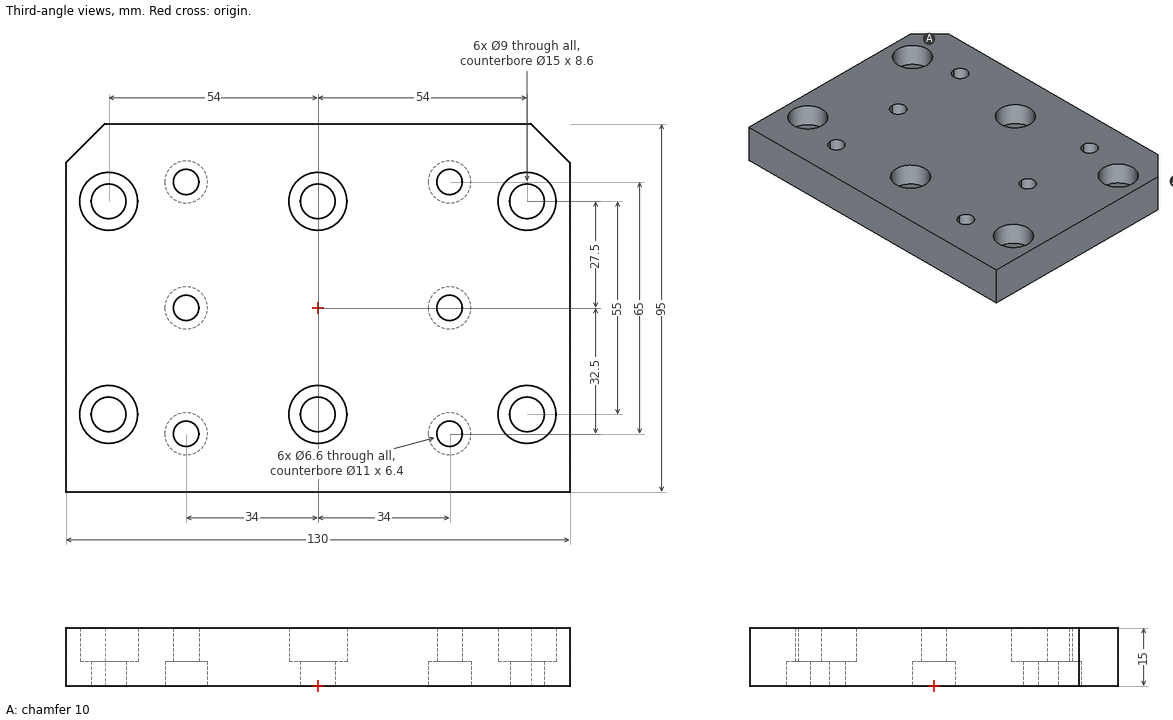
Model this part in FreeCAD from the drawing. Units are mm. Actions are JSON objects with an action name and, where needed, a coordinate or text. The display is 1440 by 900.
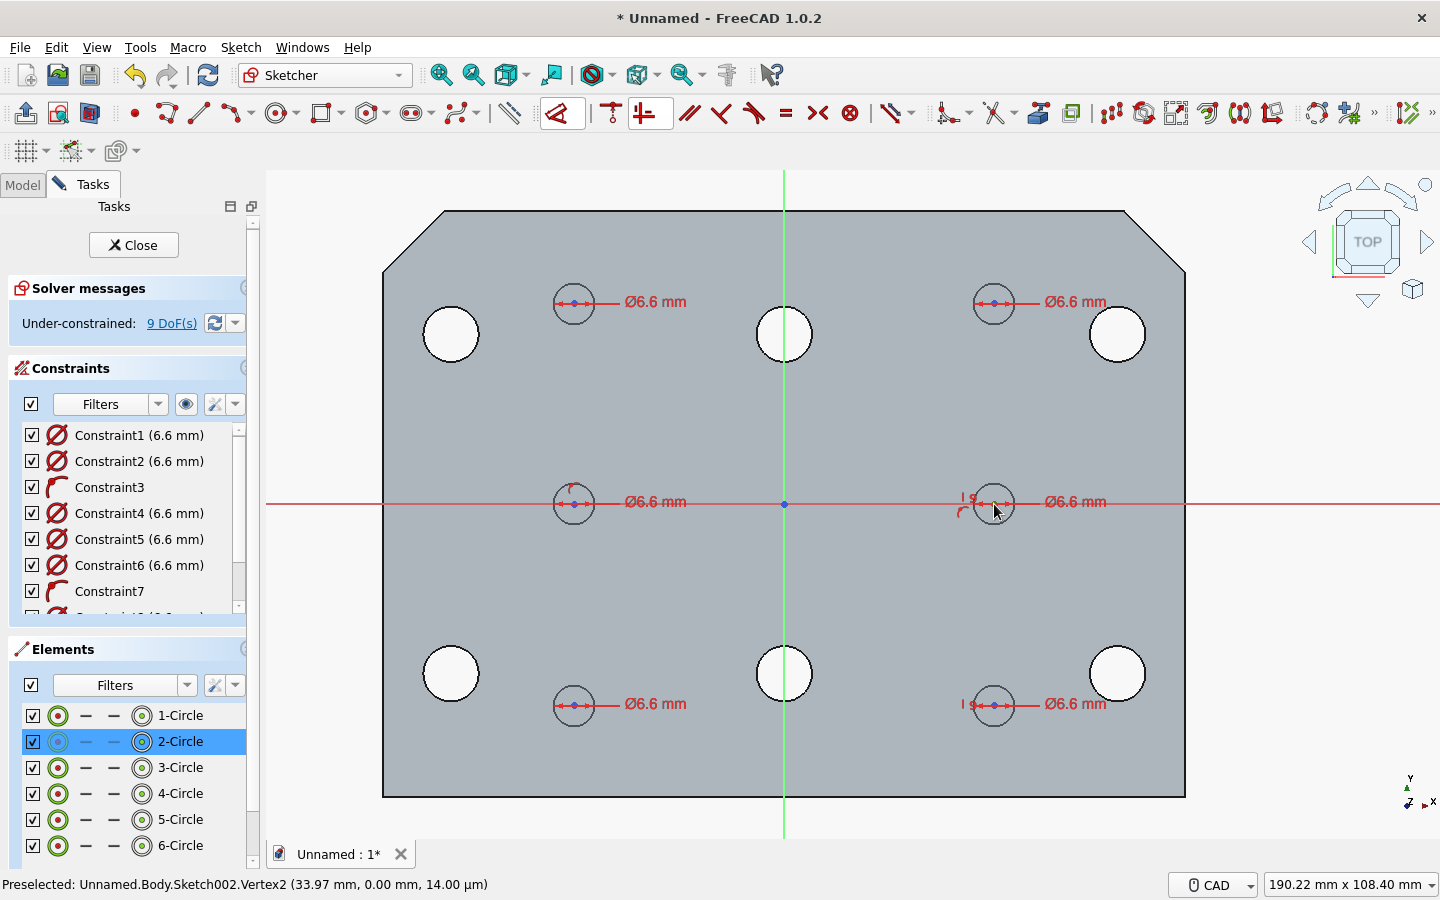
{"action": "left_click", "coordinate": [994, 304]}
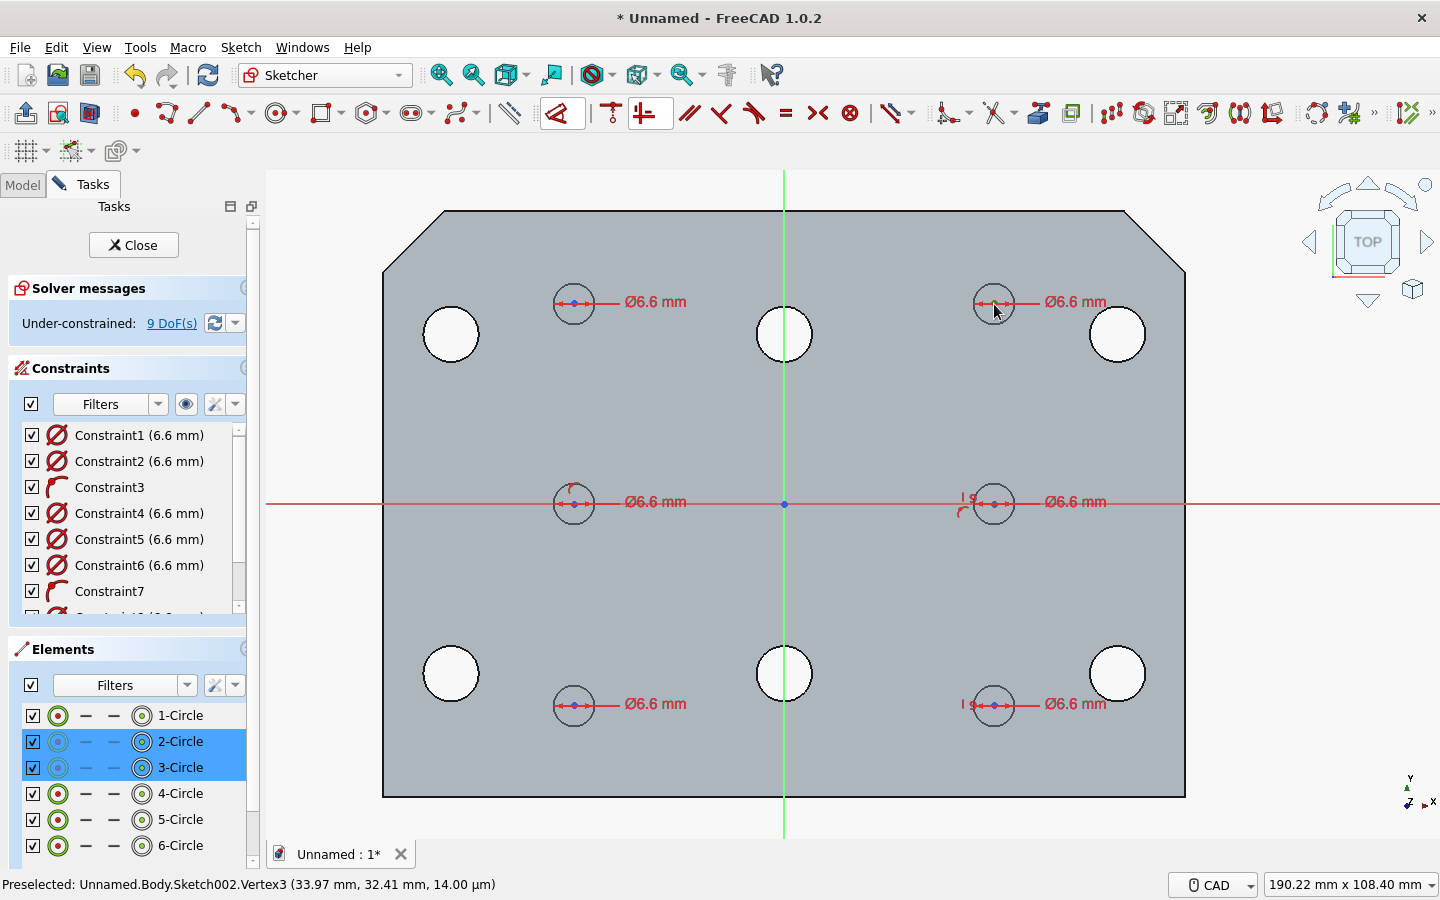
{"action": "key", "text": "v"}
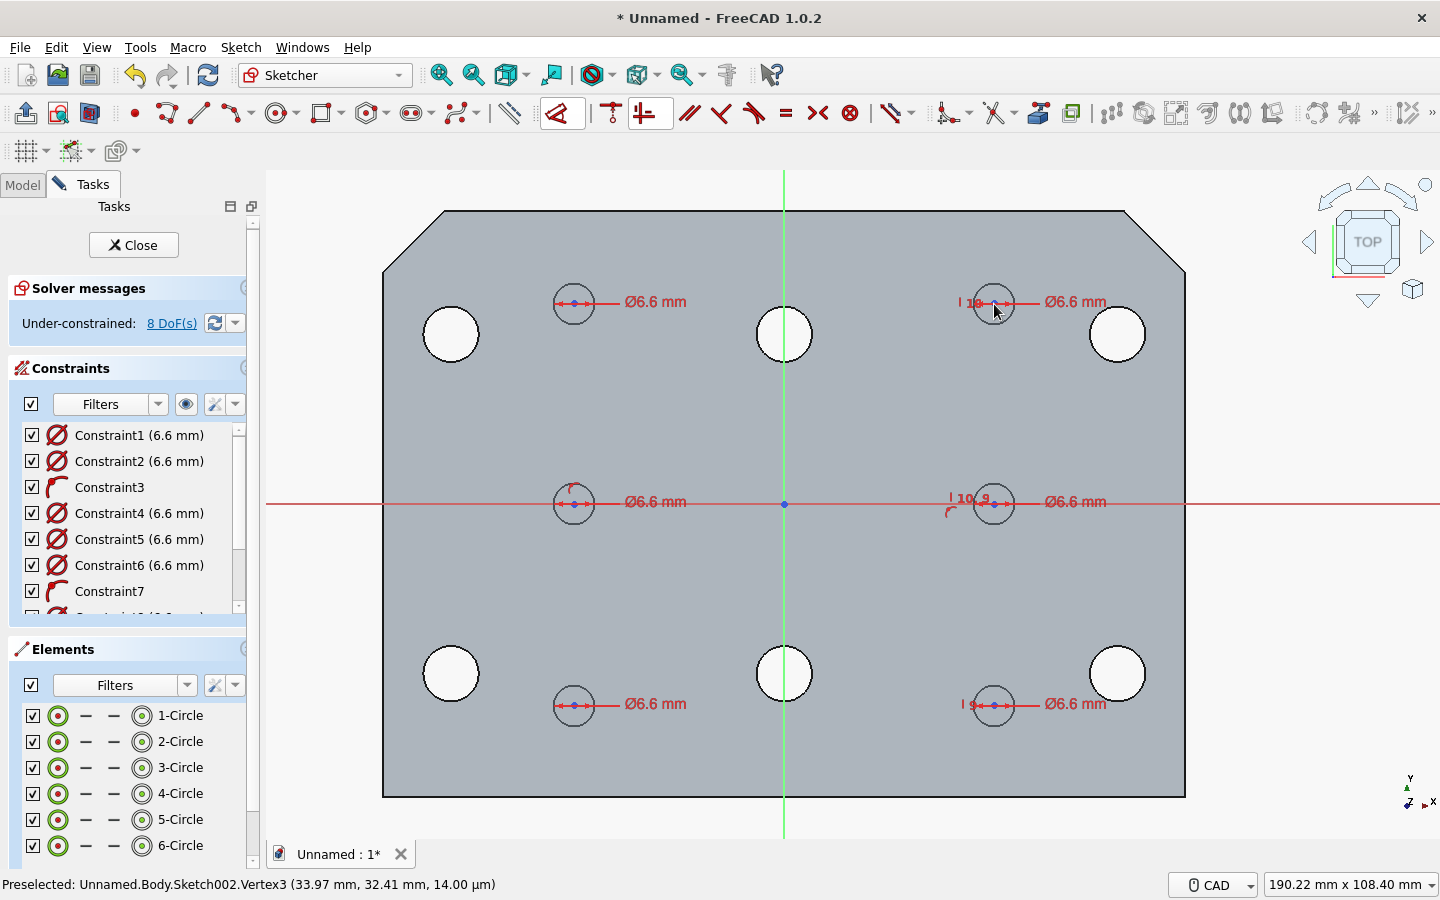
{"action": "left_click", "coordinate": [994, 706]}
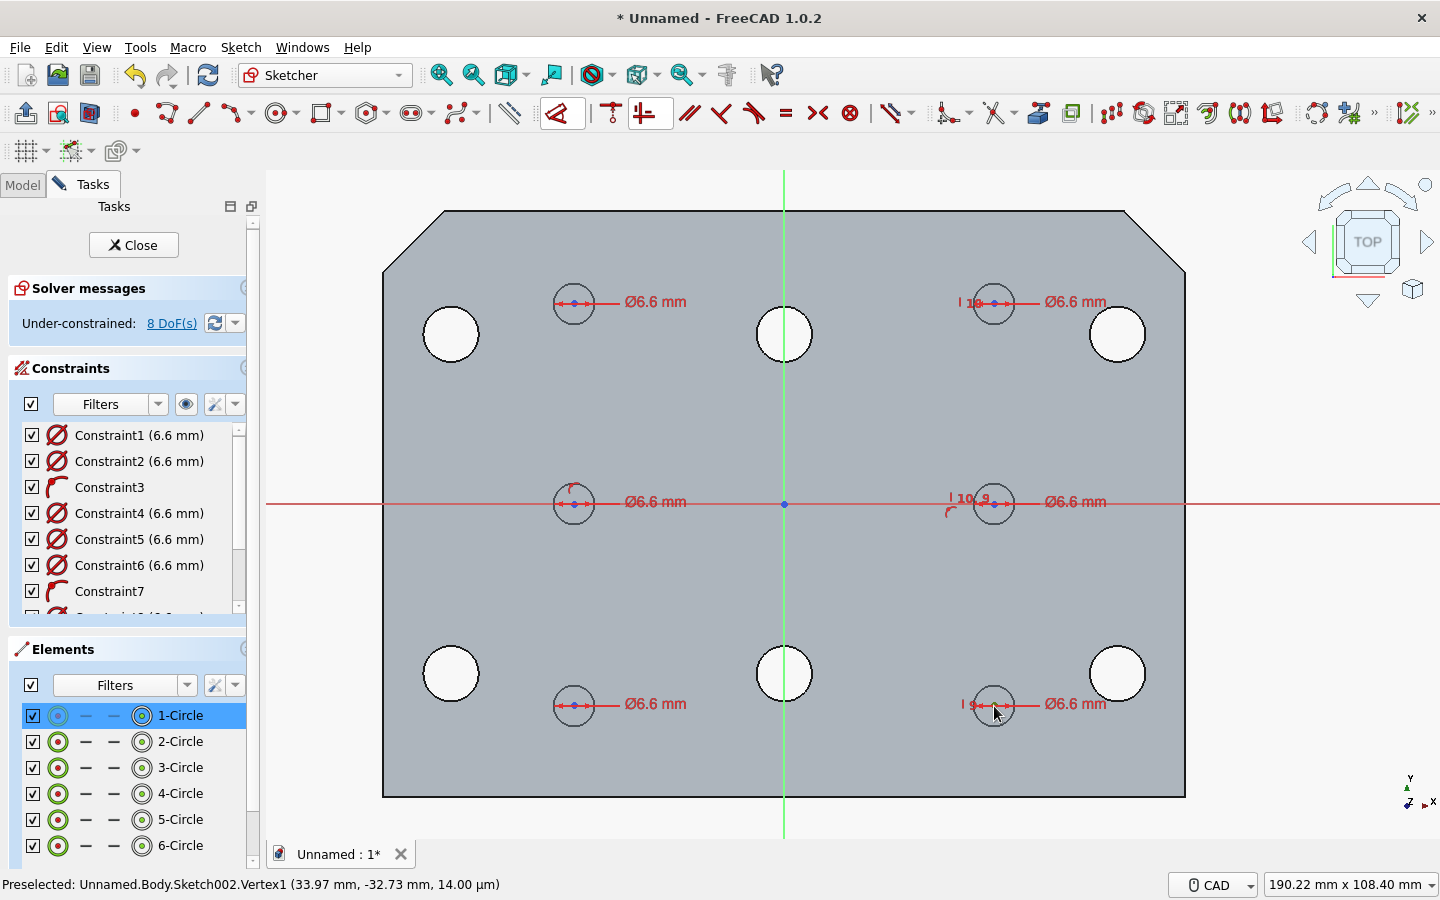
{"action": "left_click", "coordinate": [574, 706]}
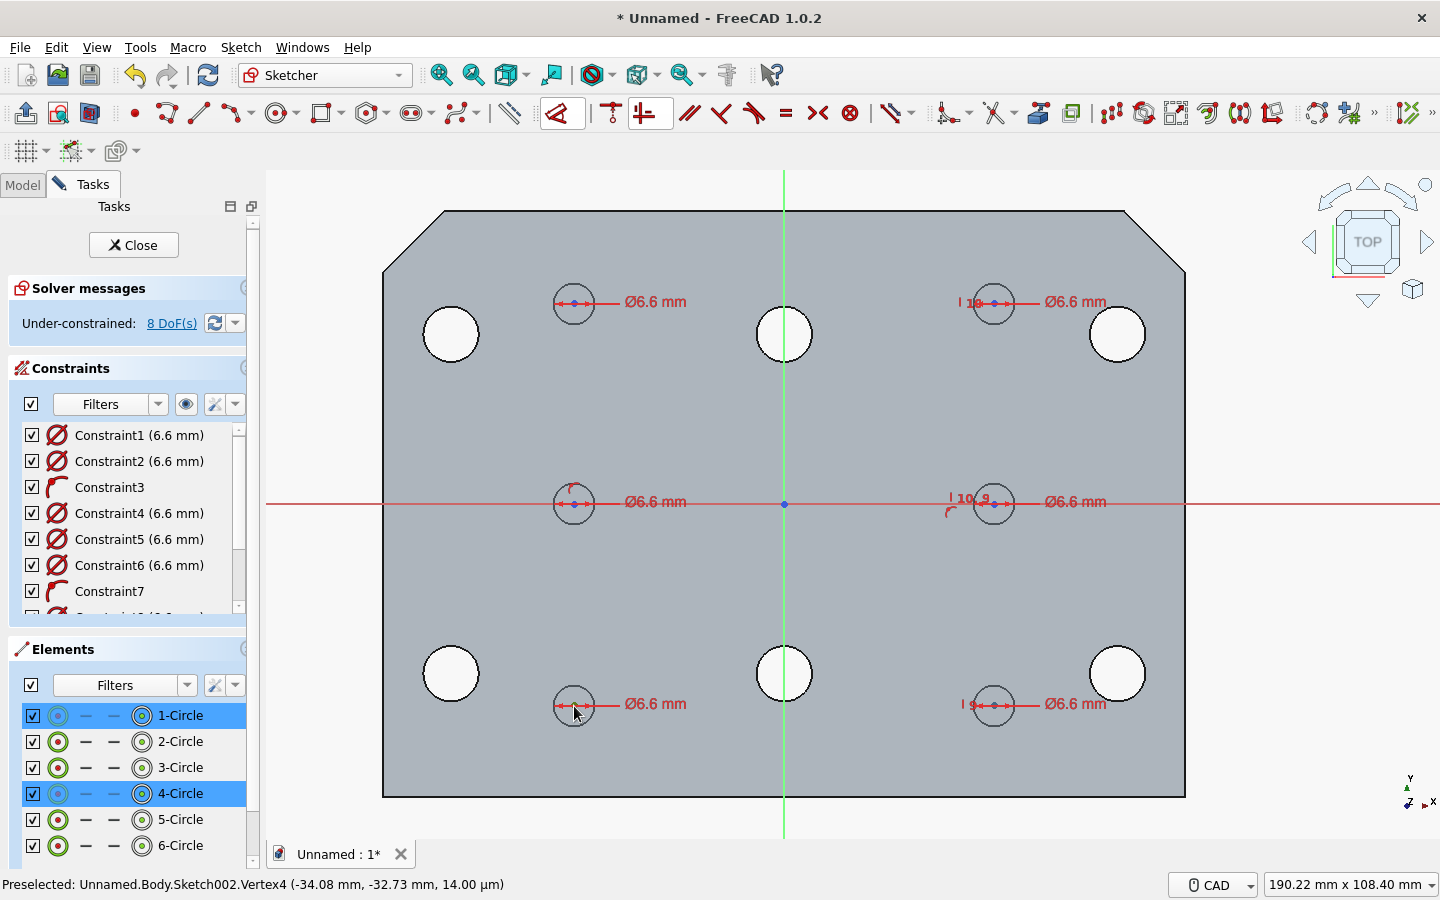
{"action": "key", "text": "h"}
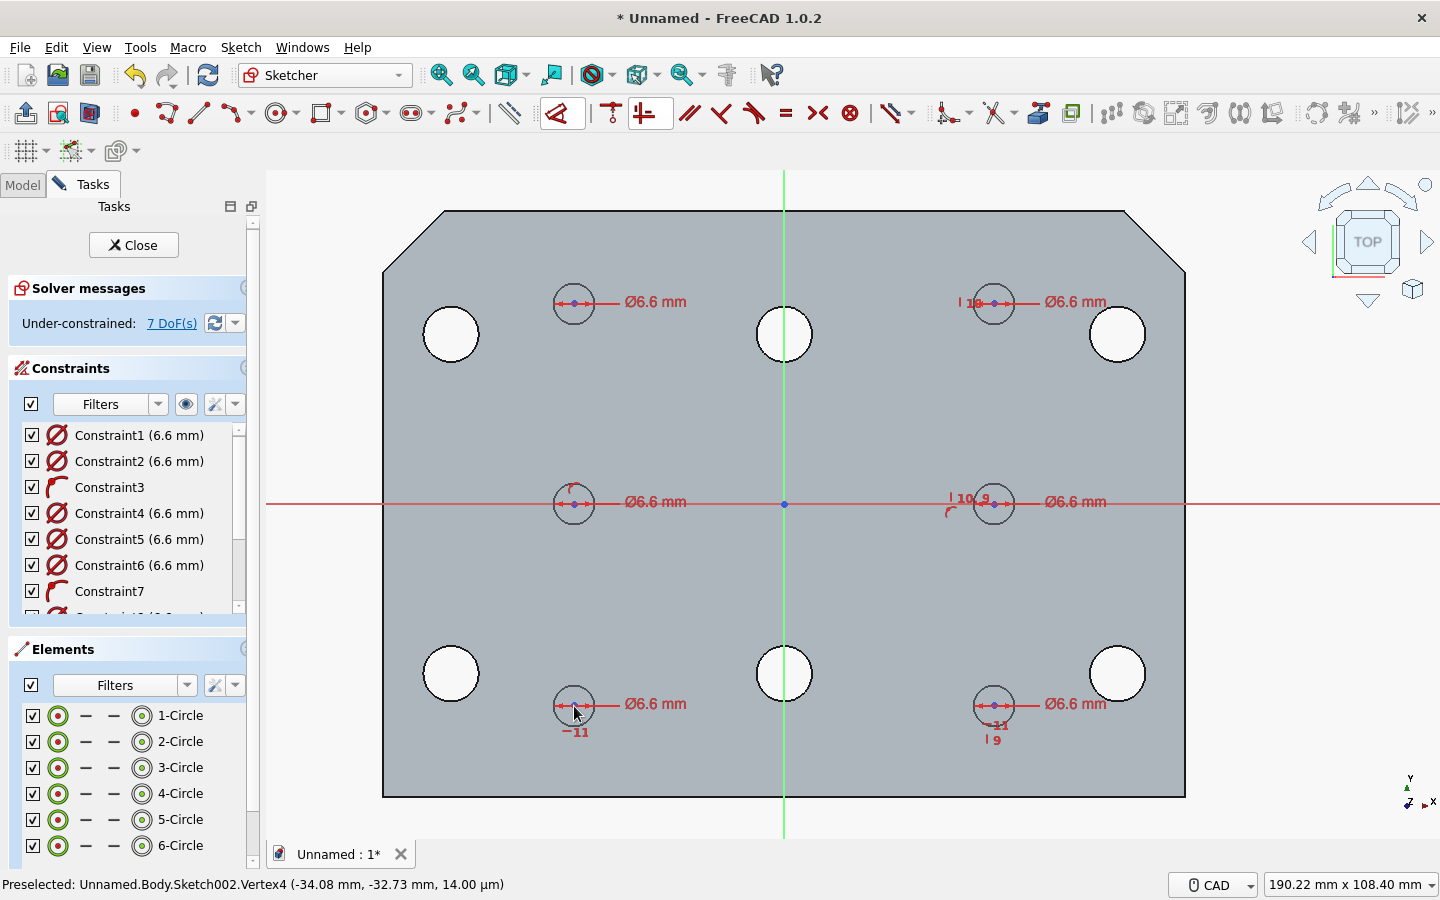
{"action": "left_click", "coordinate": [574, 706]}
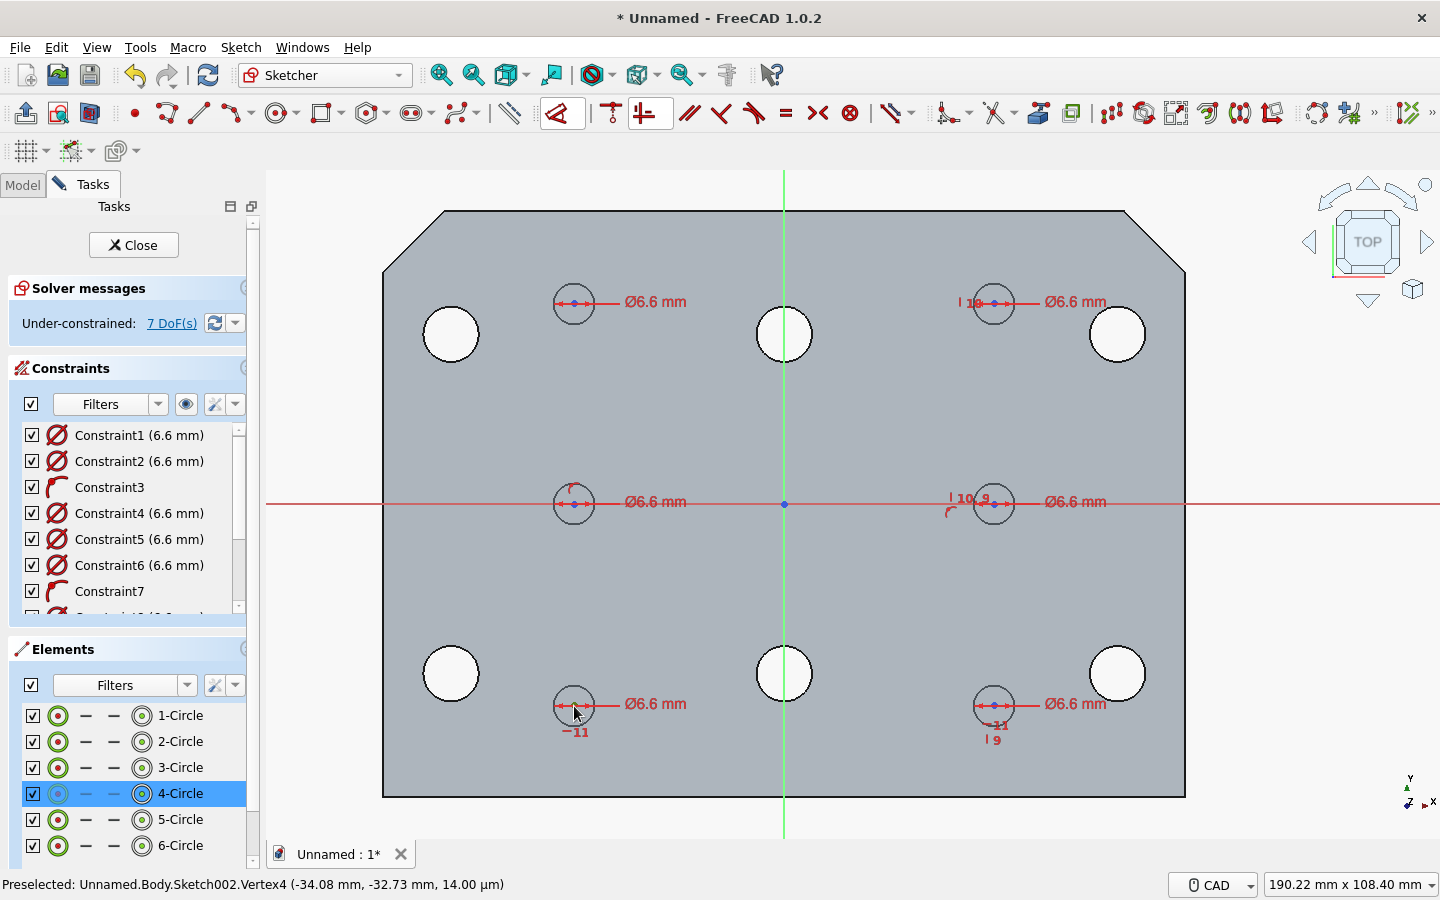
{"action": "left_click", "coordinate": [574, 504]}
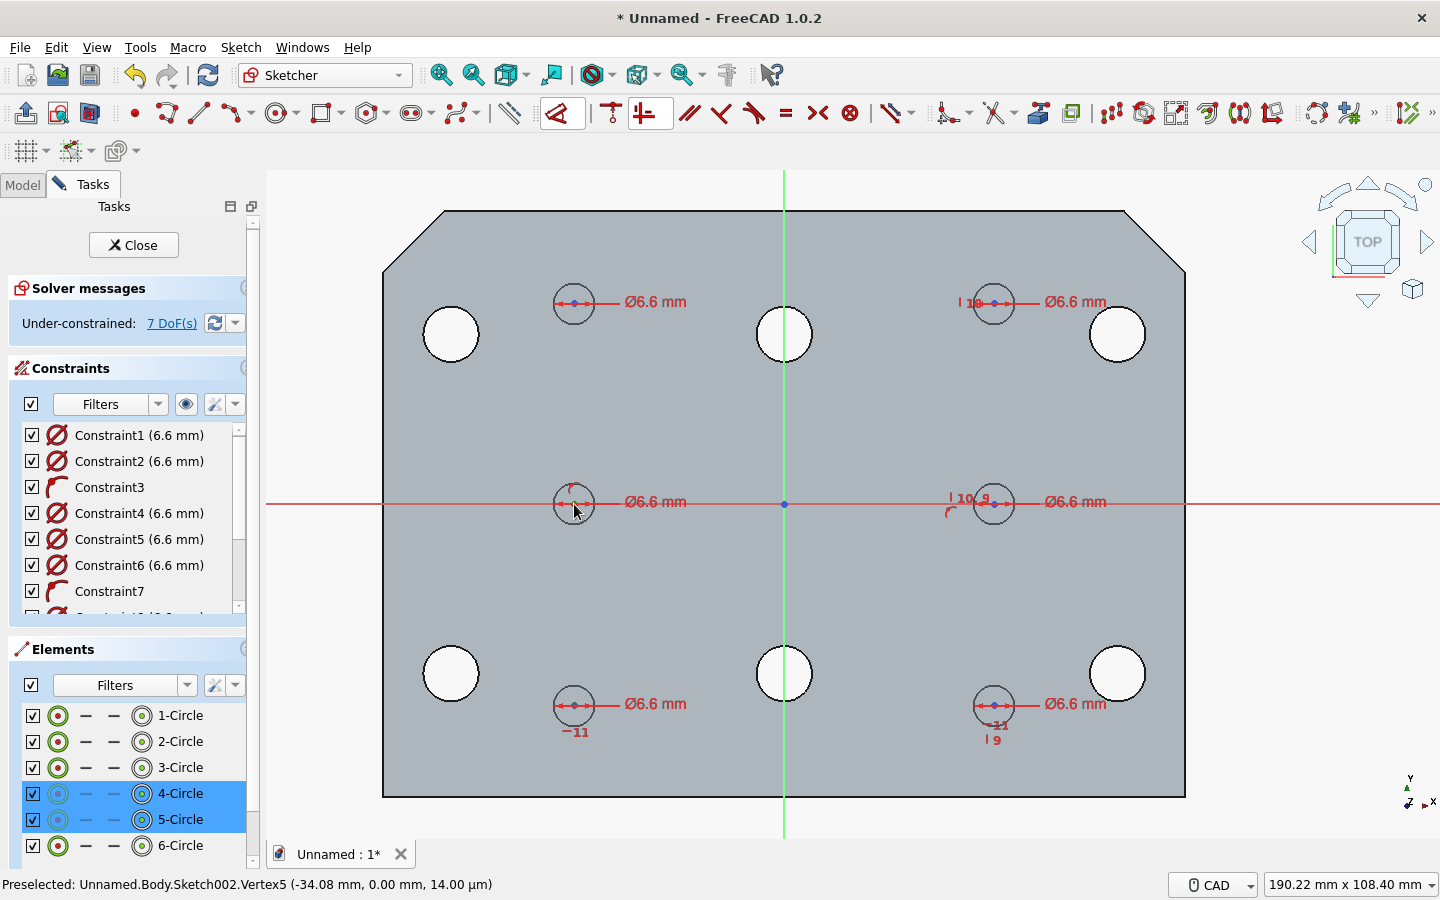
{"action": "left_click", "coordinate": [668, 114]}